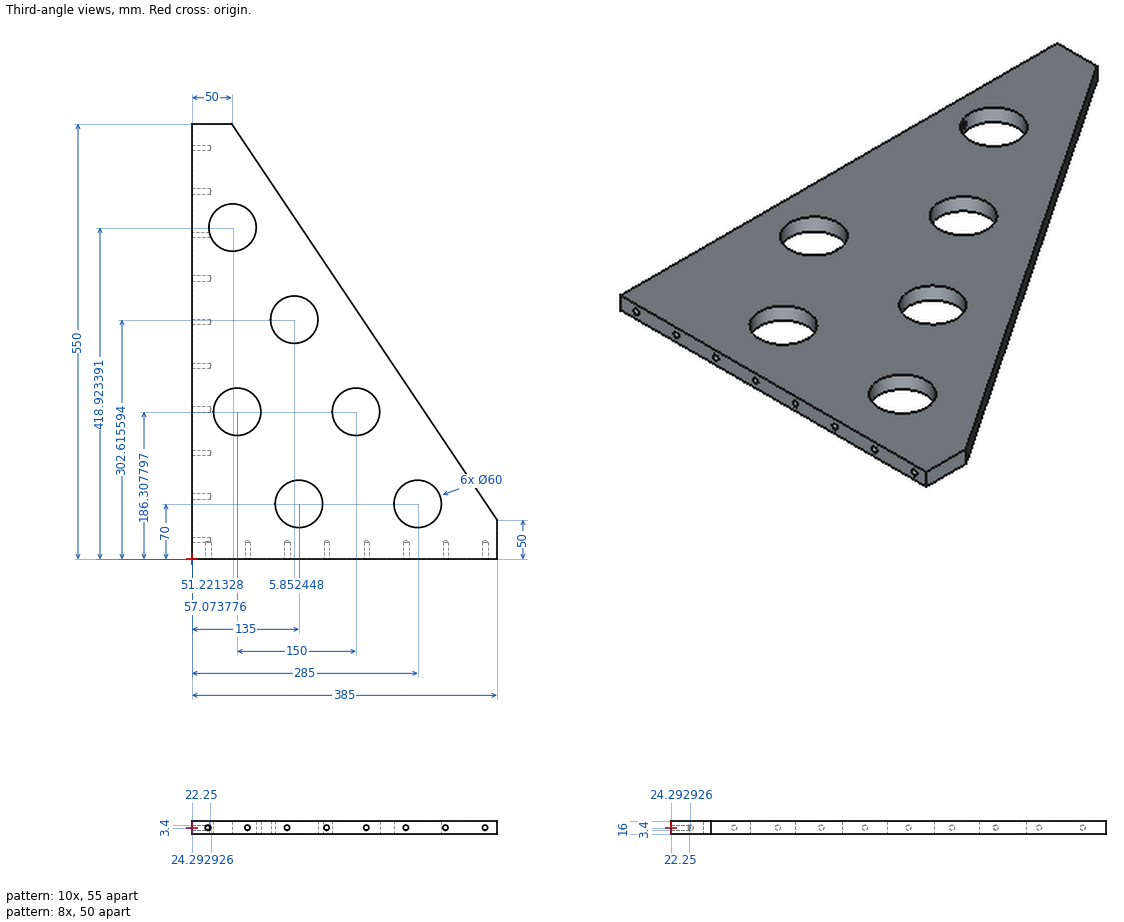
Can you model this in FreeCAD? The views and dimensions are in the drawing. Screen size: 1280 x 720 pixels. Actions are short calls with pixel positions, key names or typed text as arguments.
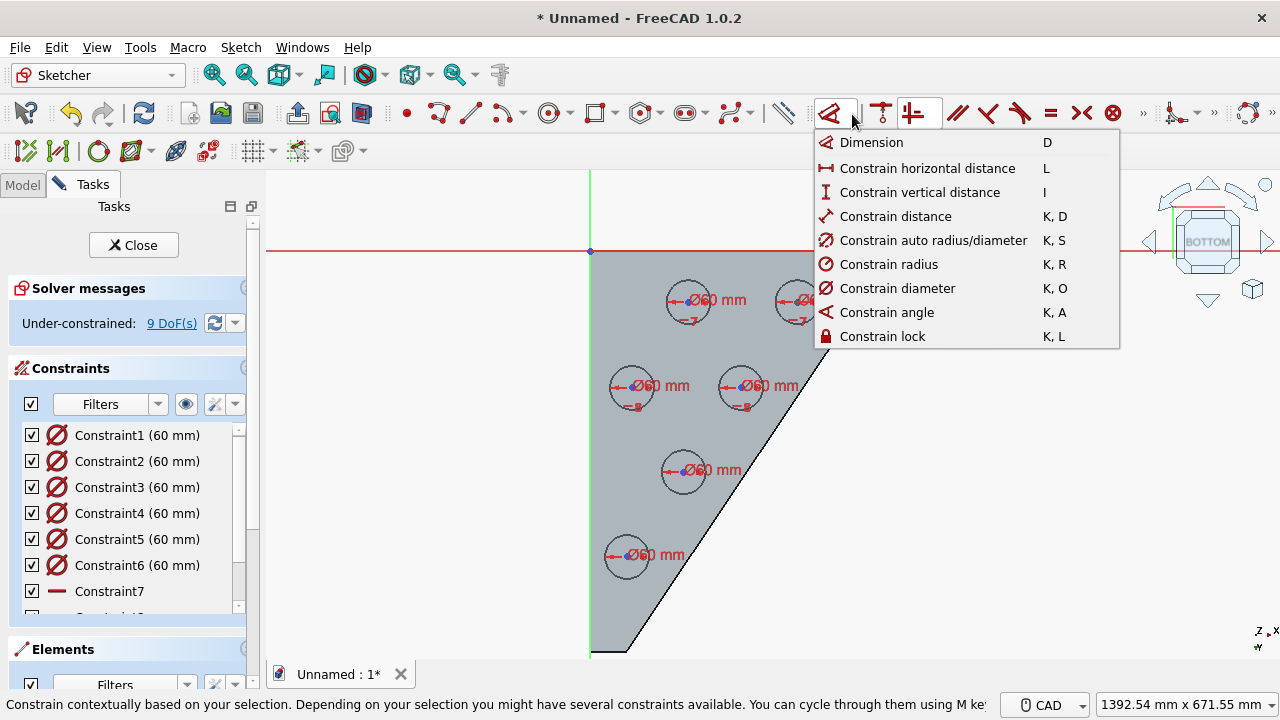
click(967, 168)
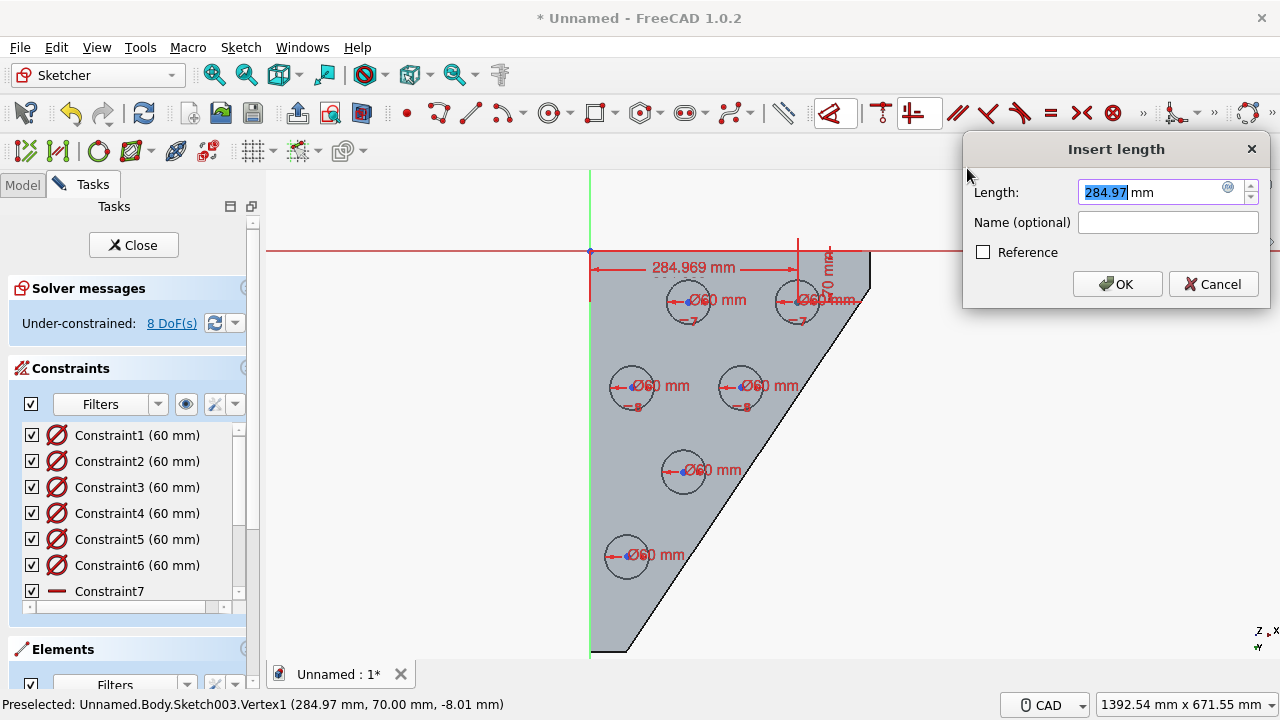
text(285)
key(Return)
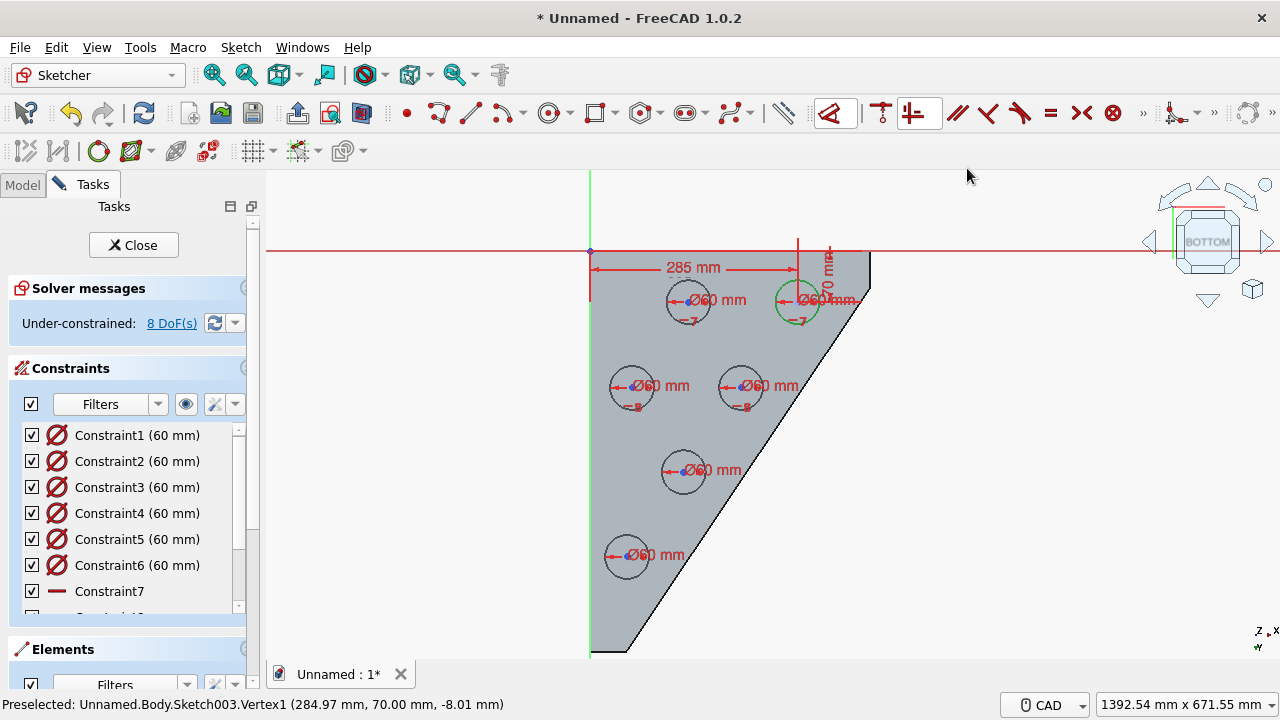
click(689, 302)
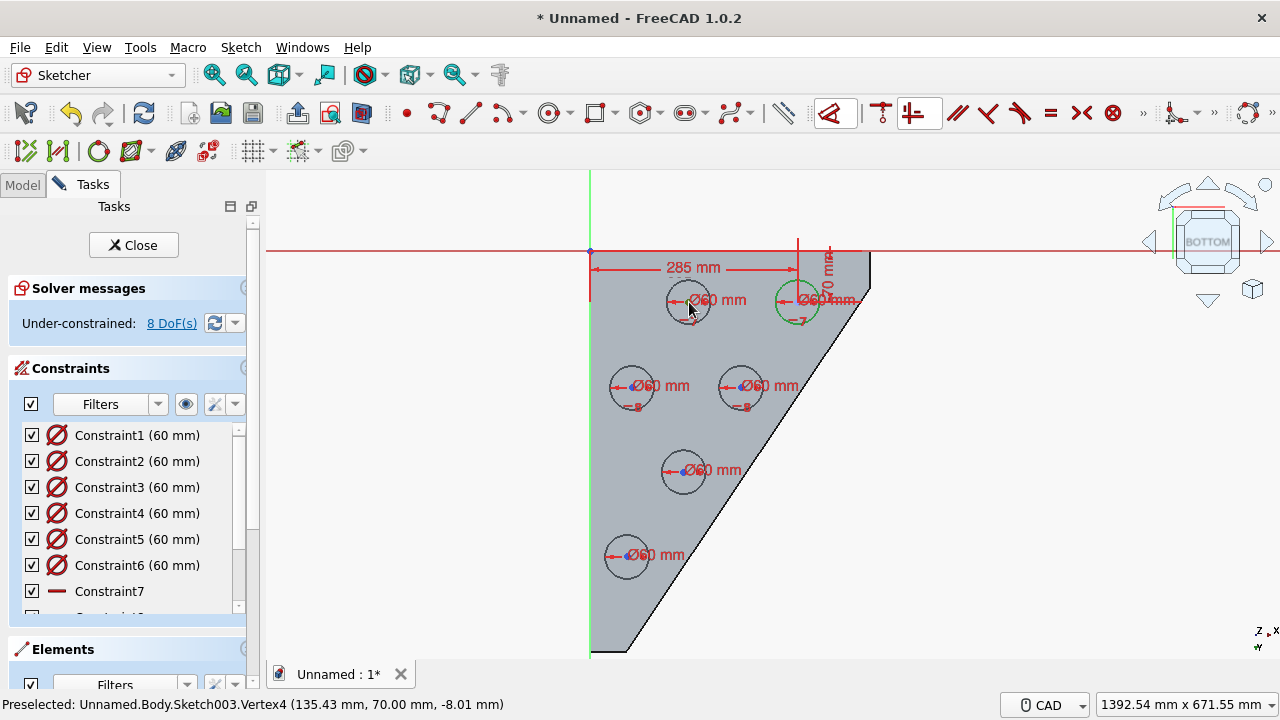
click(852, 114)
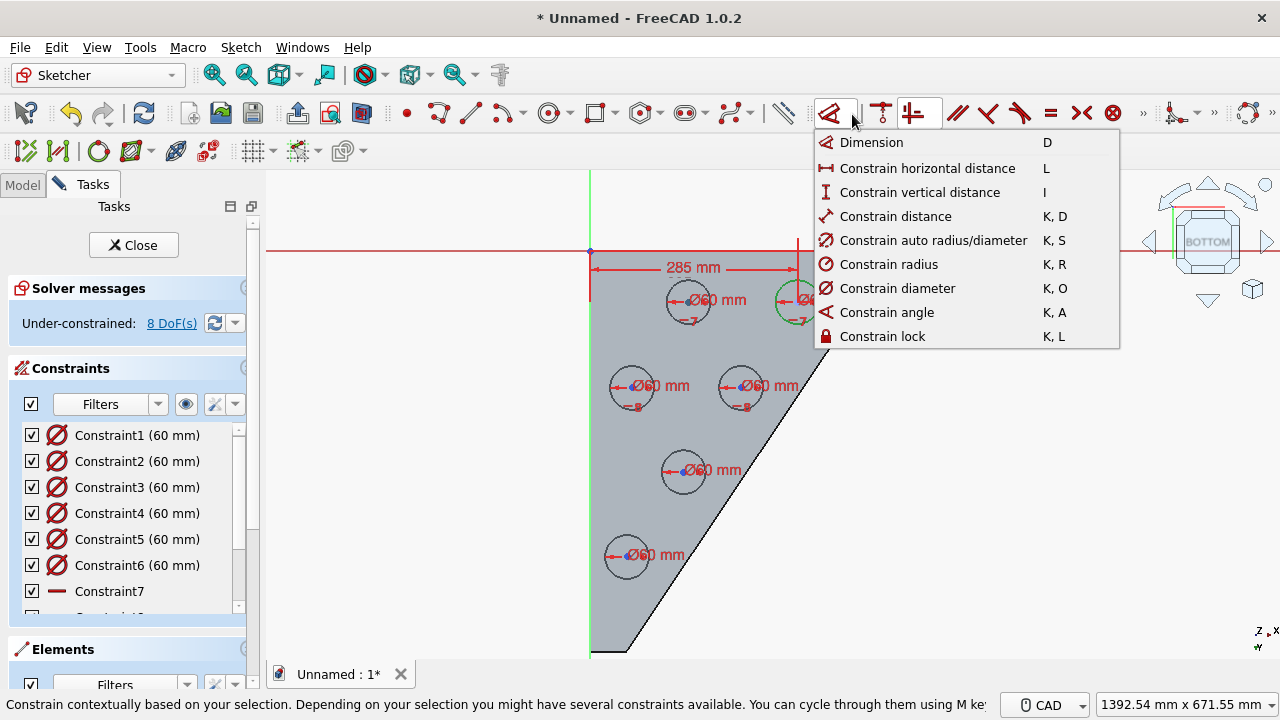
click(967, 168)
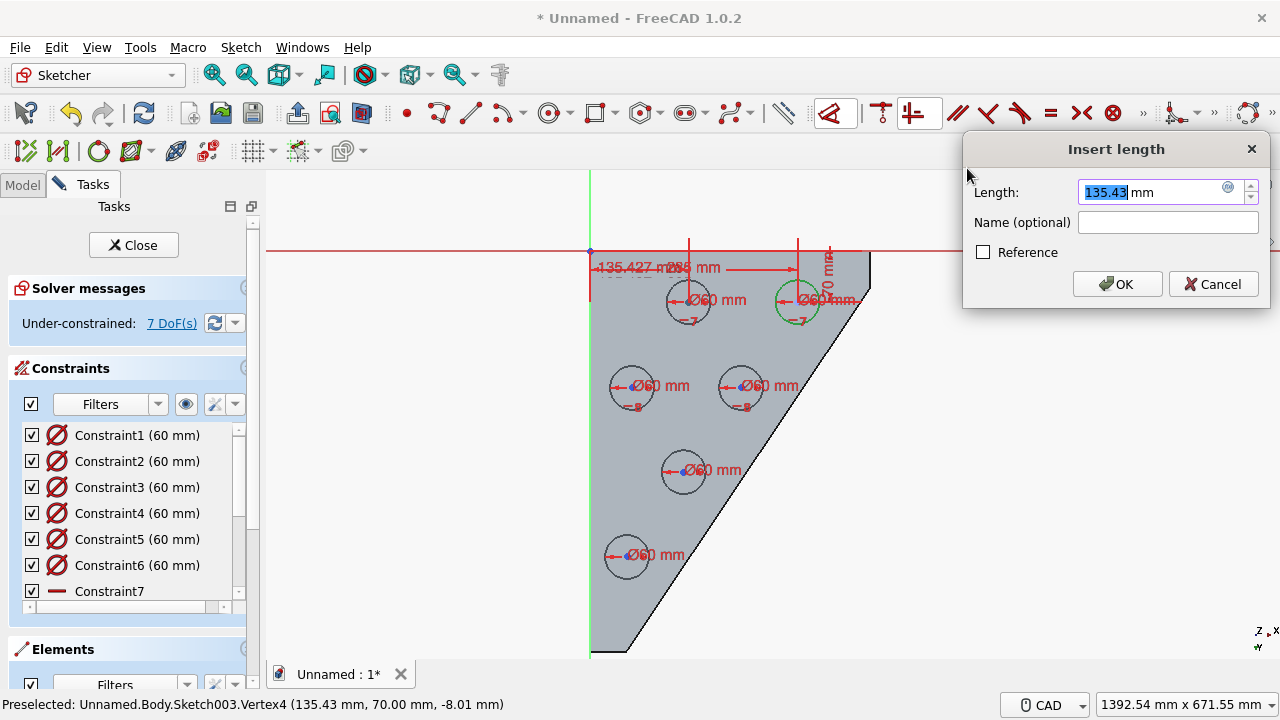
text(135)
key(Return)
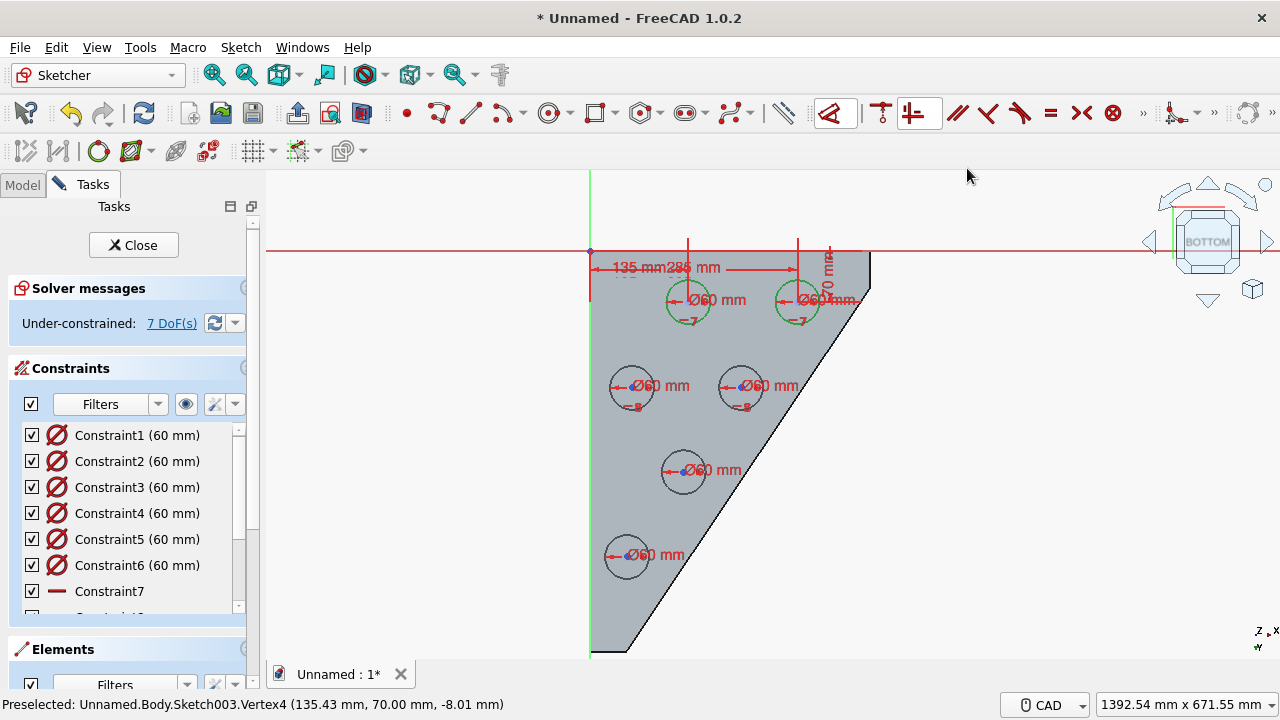
click(741, 388)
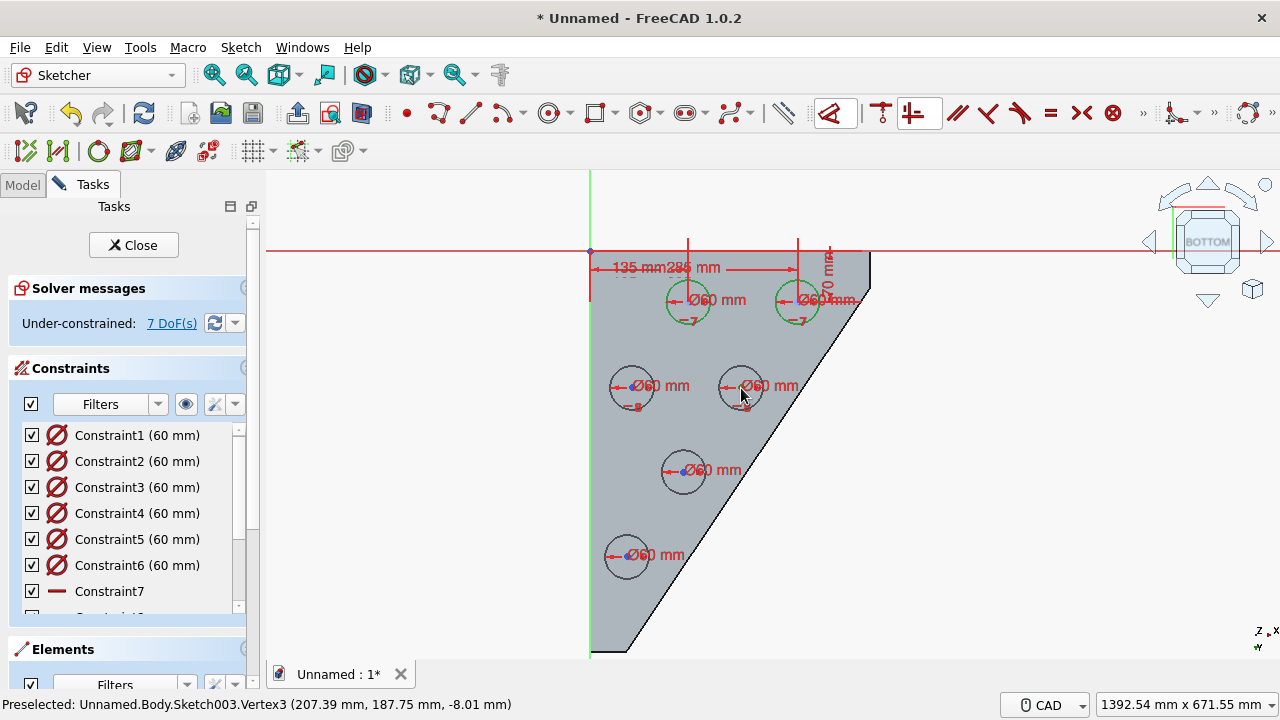
click(632, 388)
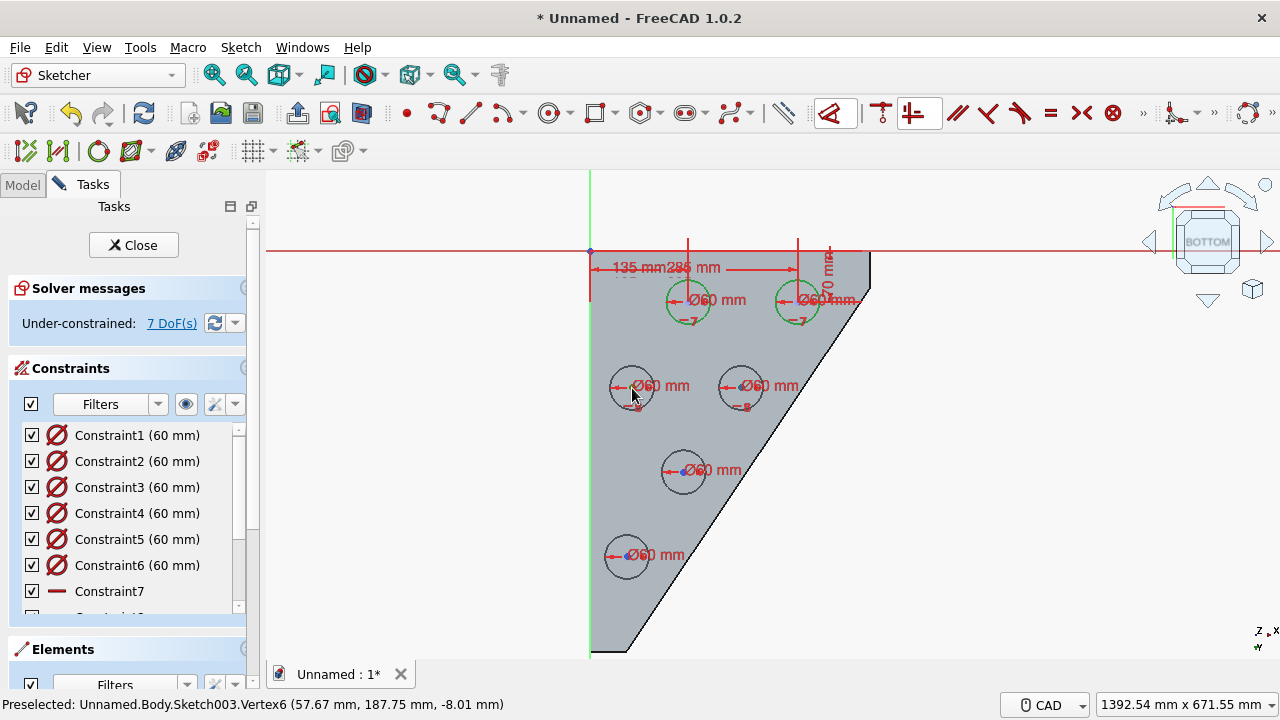
click(852, 114)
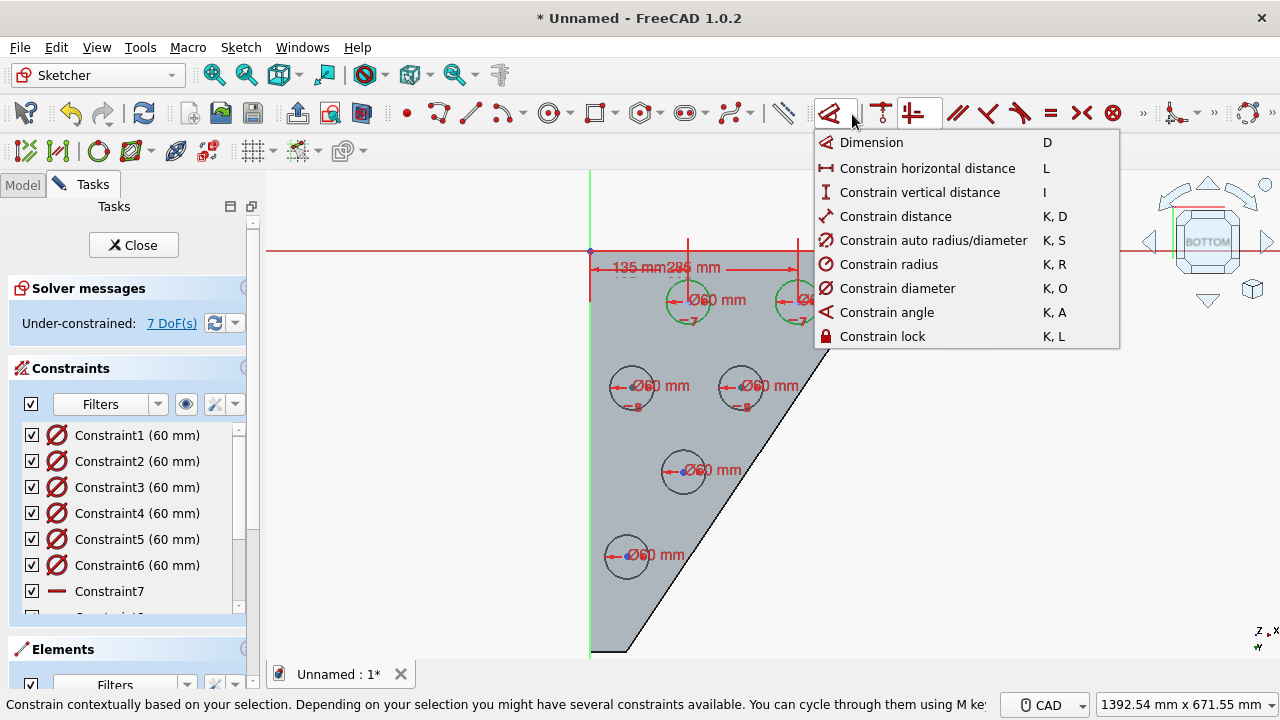
click(967, 168)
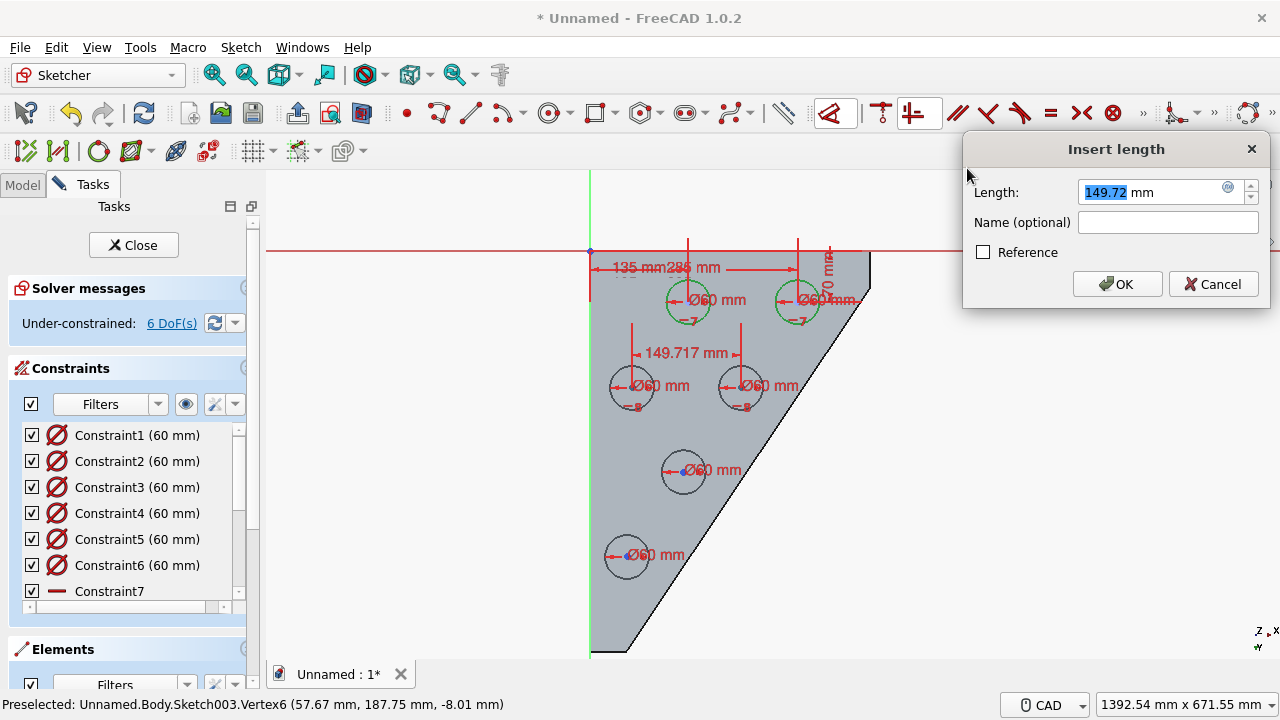
text(150)
key(Return)